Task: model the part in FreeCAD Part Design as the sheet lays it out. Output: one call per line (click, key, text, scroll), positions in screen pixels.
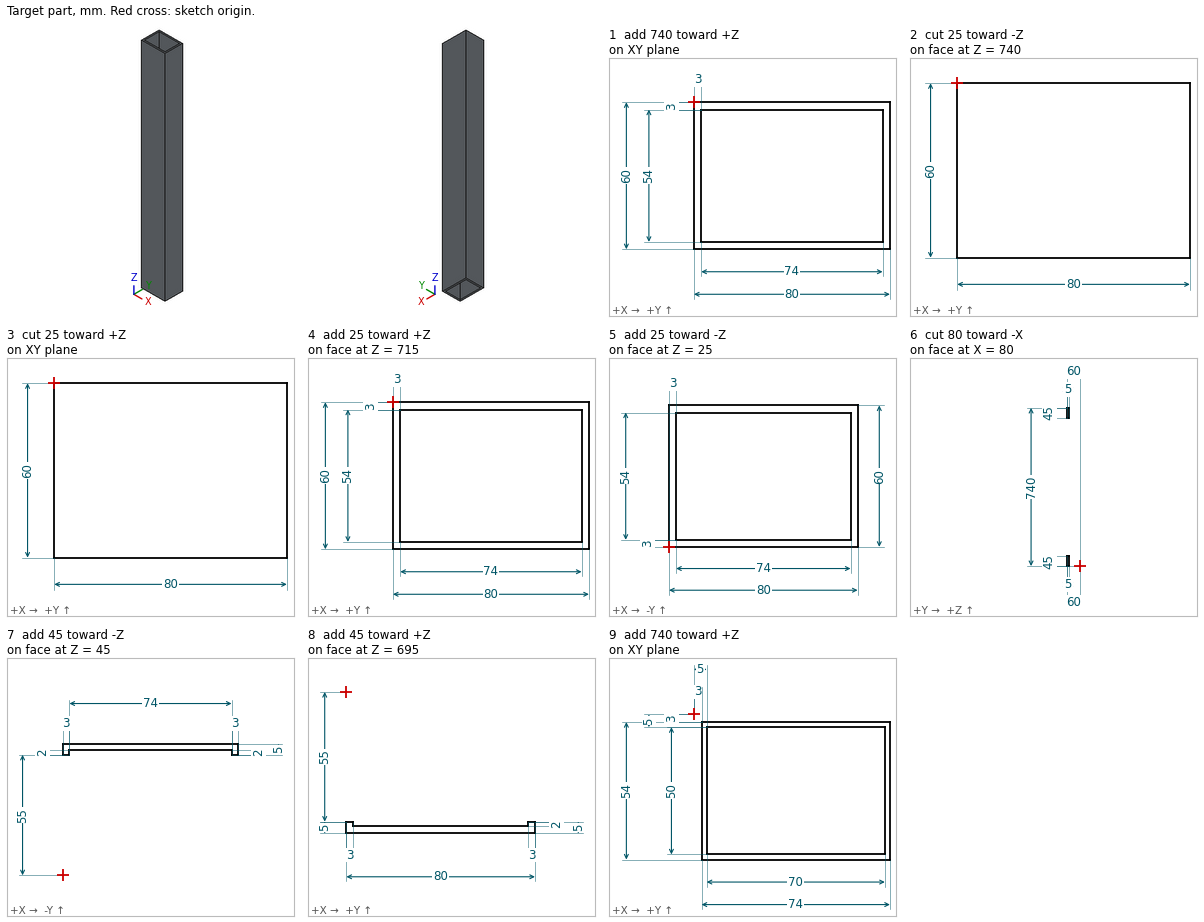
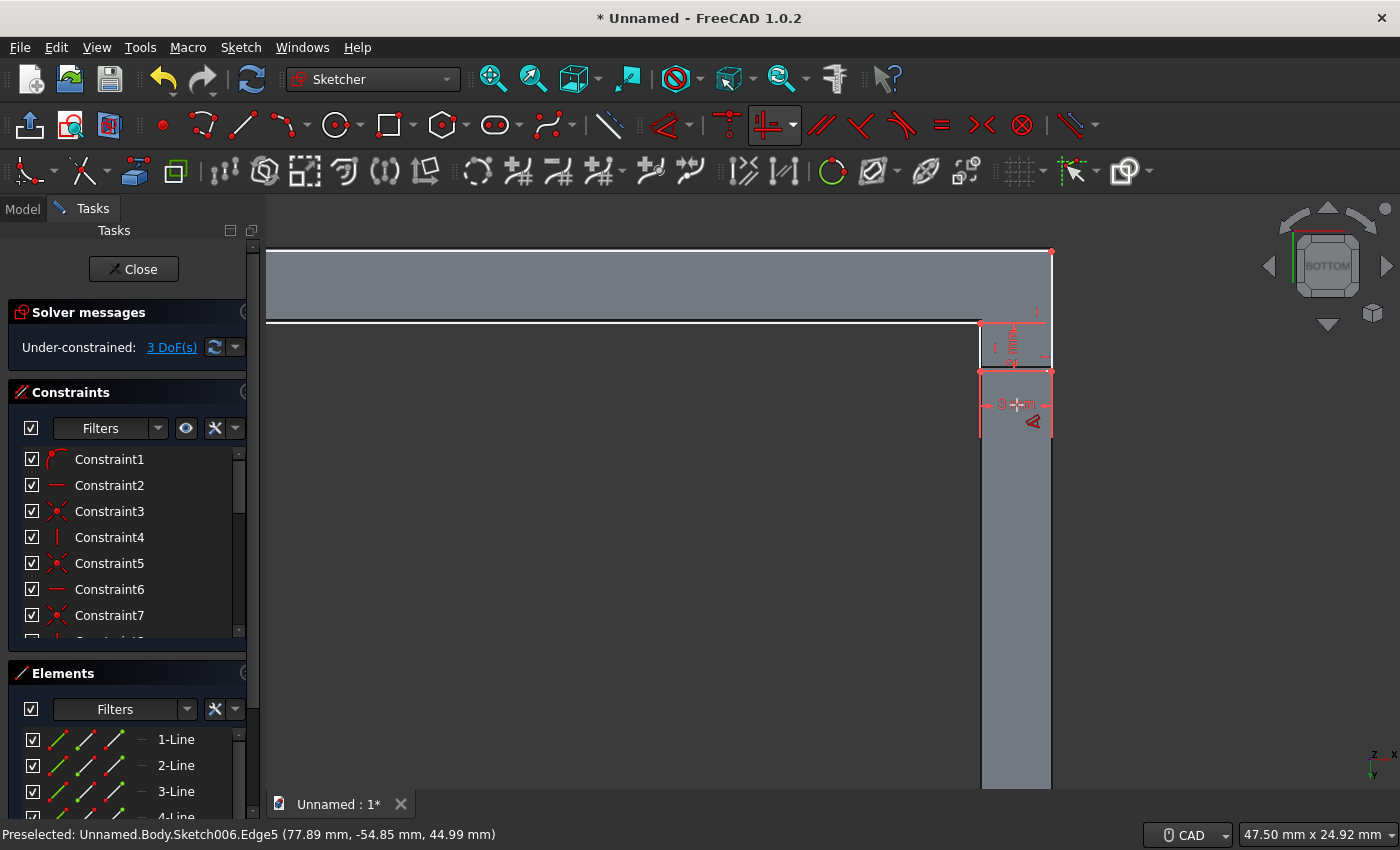
click(1052, 335)
click(1086, 311)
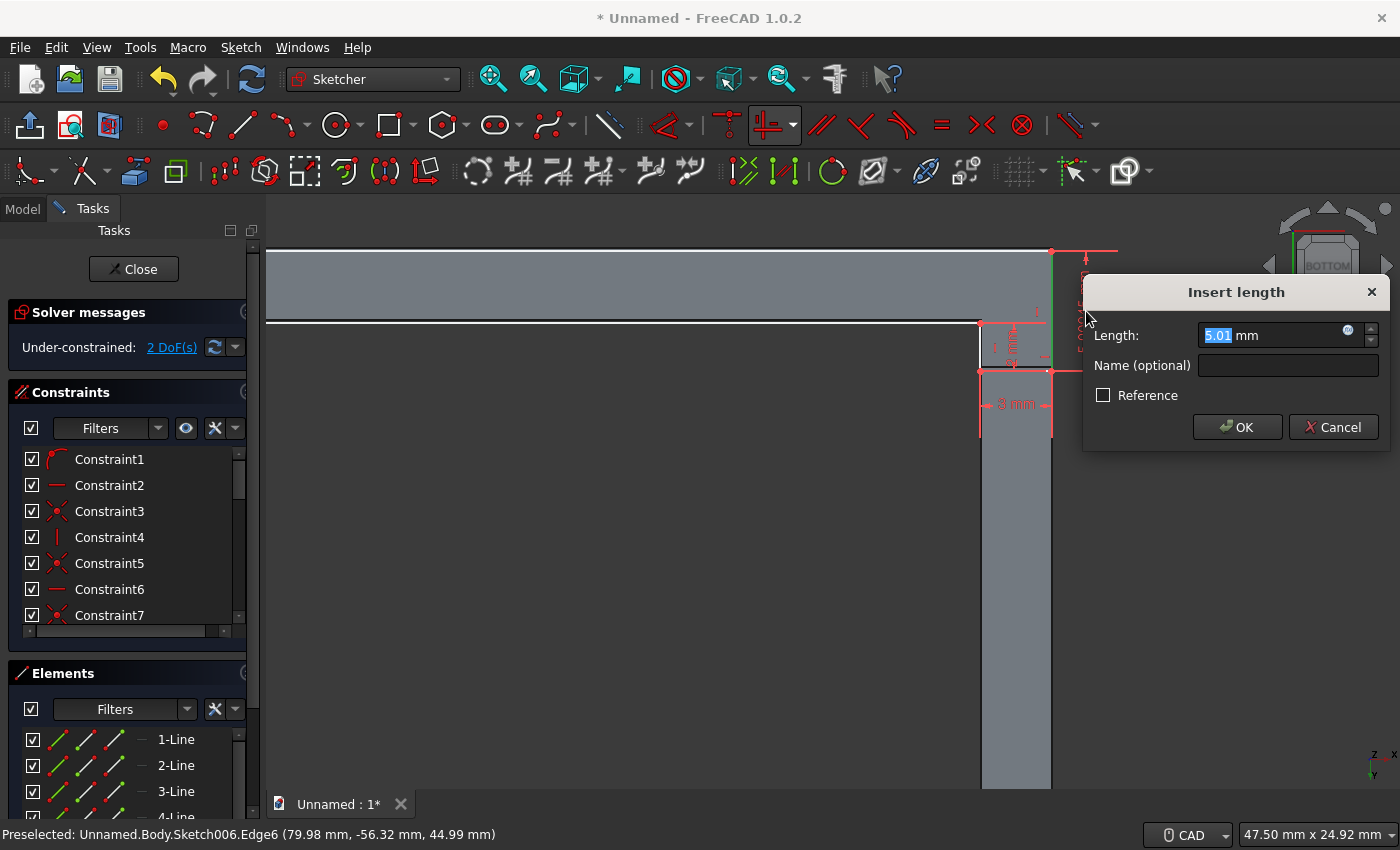
text(5)
key(Return)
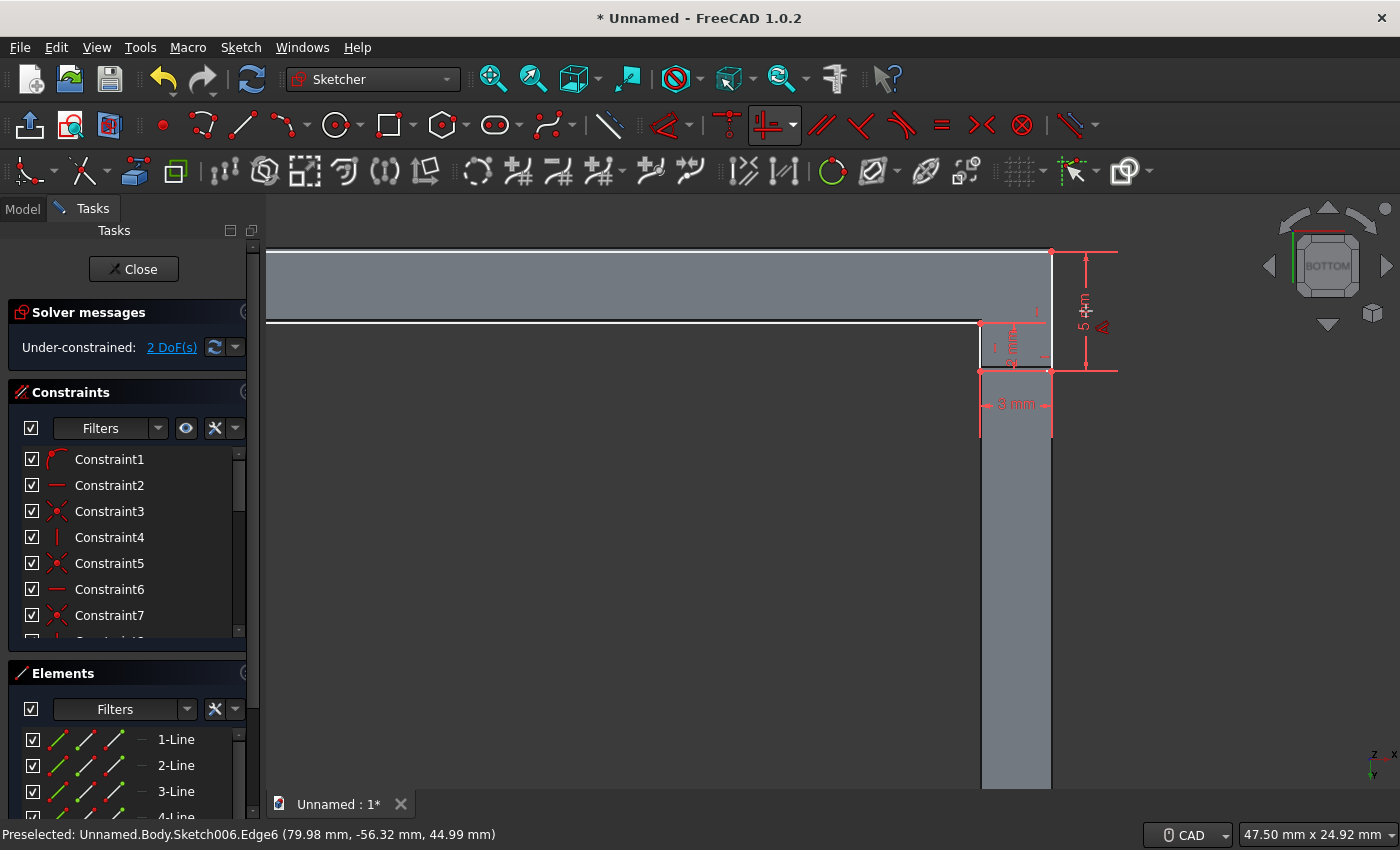
scroll(983, 337, down, 7)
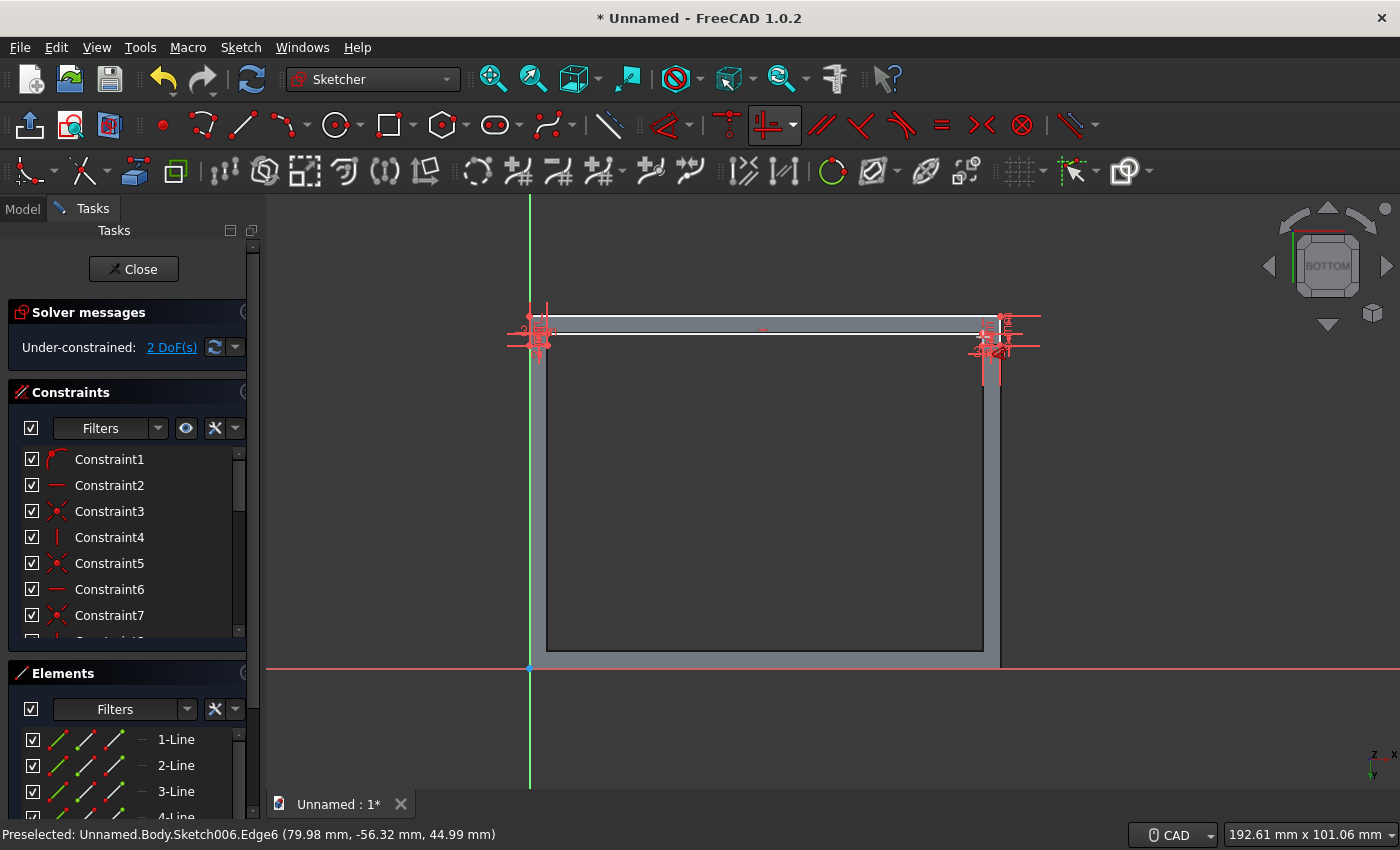
click(852, 334)
click(765, 300)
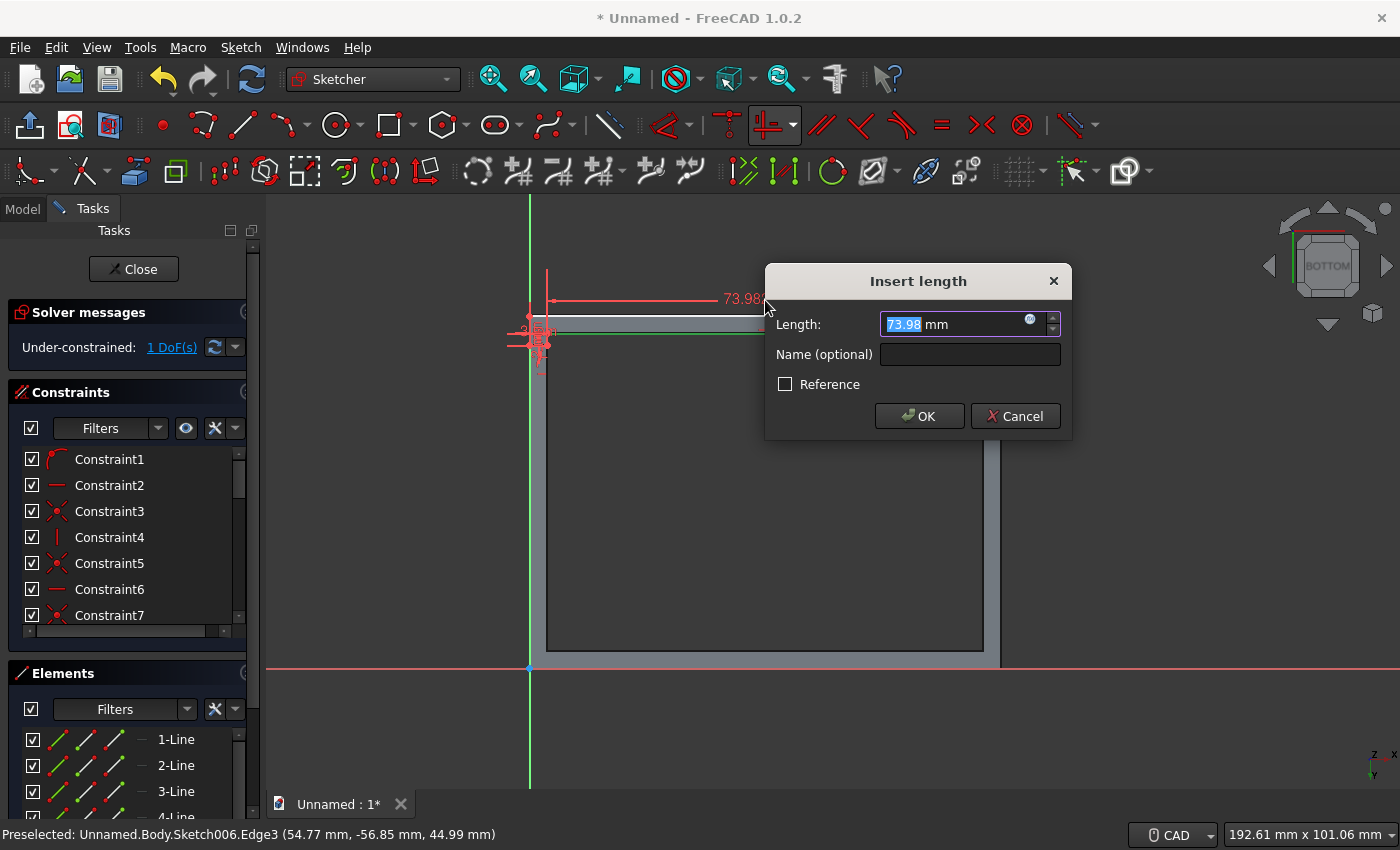
text(74)
key(Return)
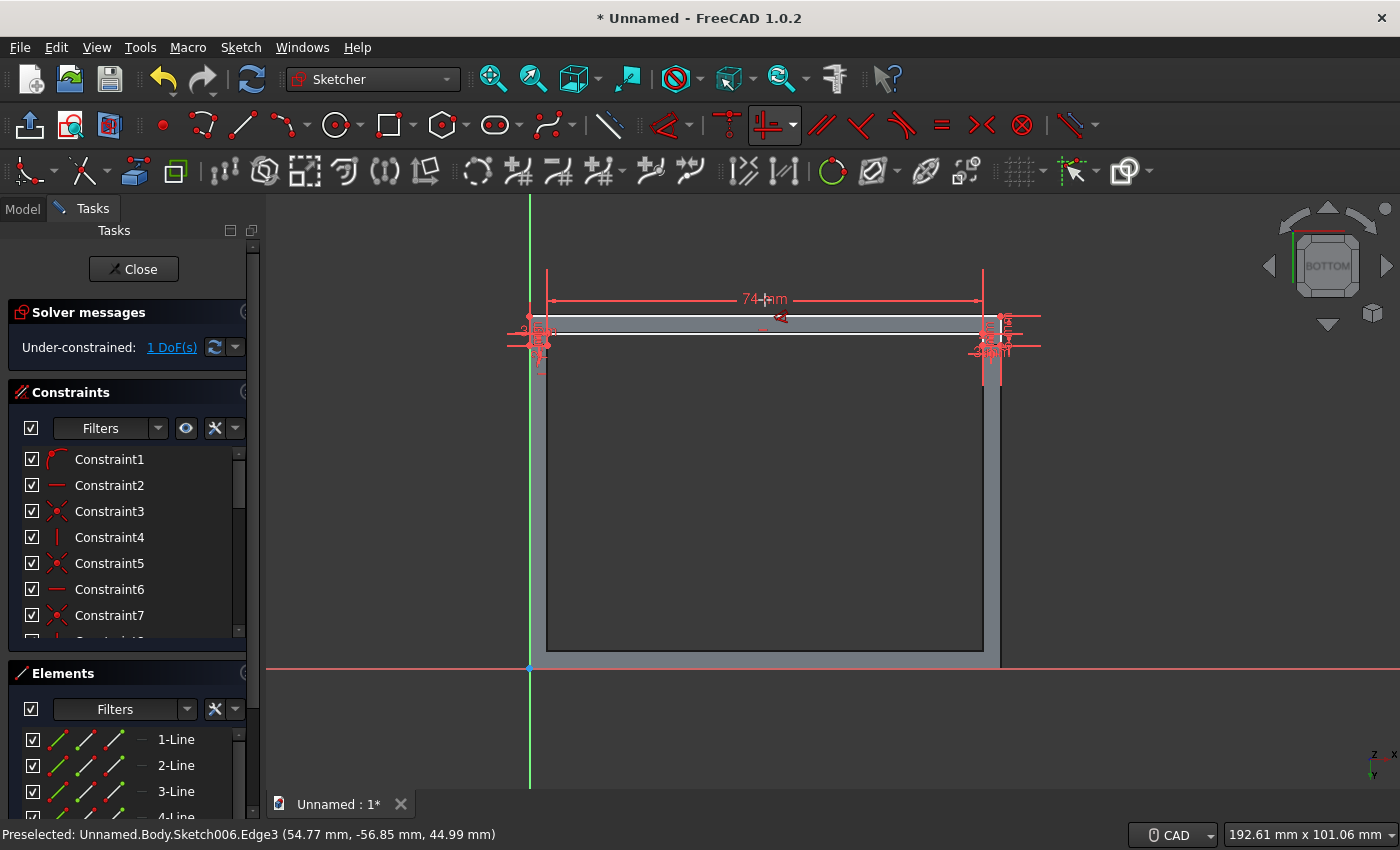
click(530, 346)
click(496, 507)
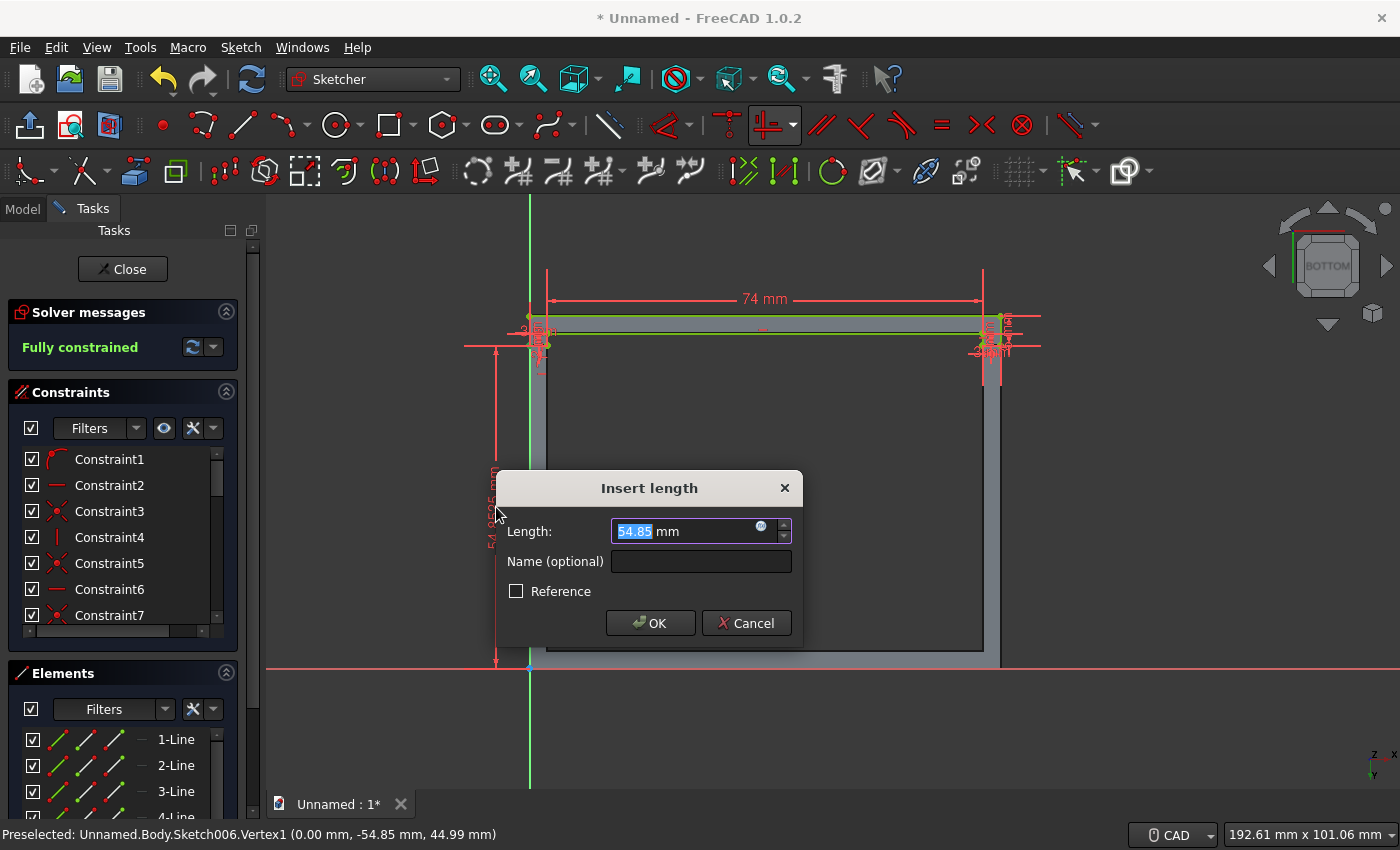
text(55)
key(Return)
key(Escape)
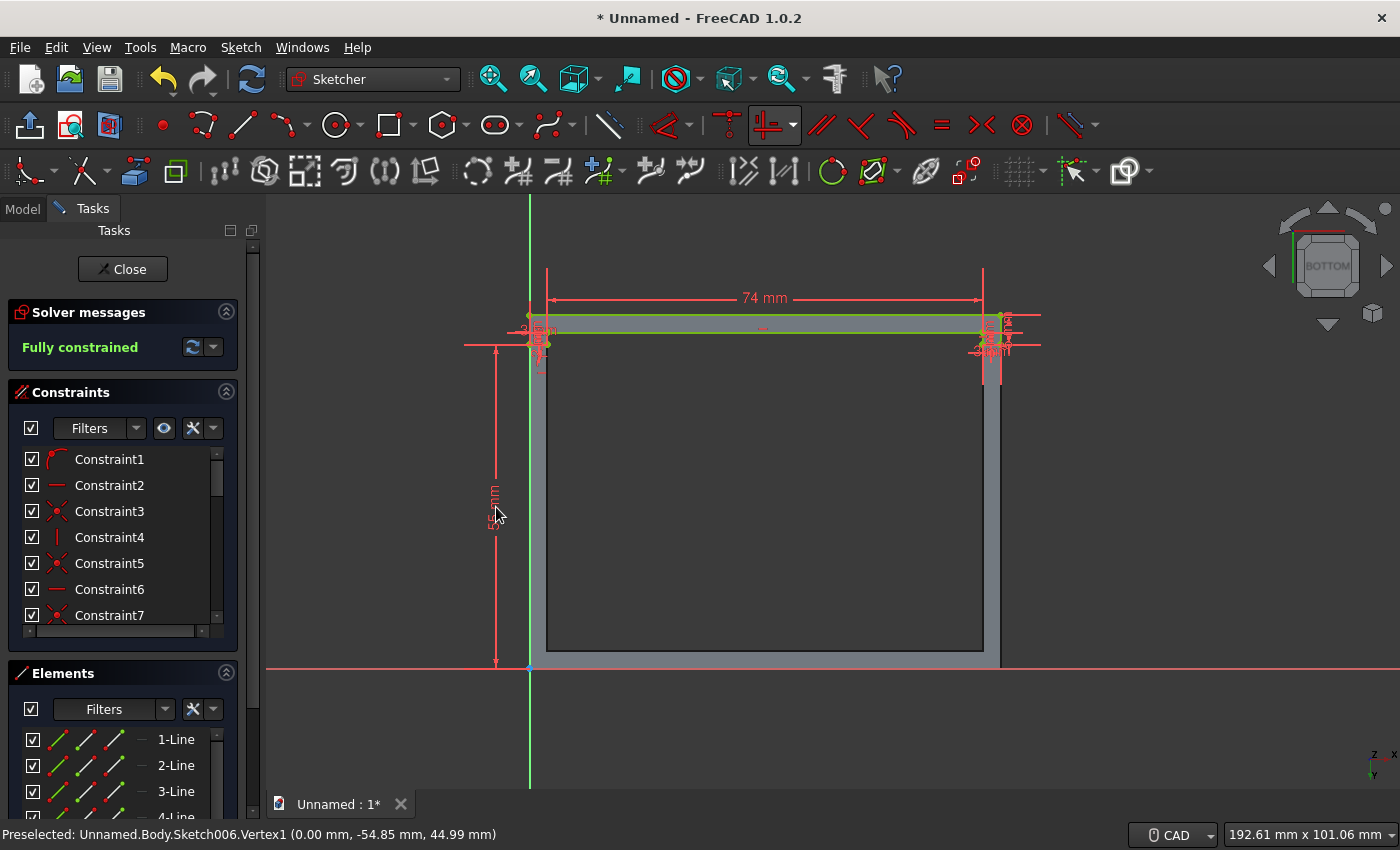
click(123, 269)